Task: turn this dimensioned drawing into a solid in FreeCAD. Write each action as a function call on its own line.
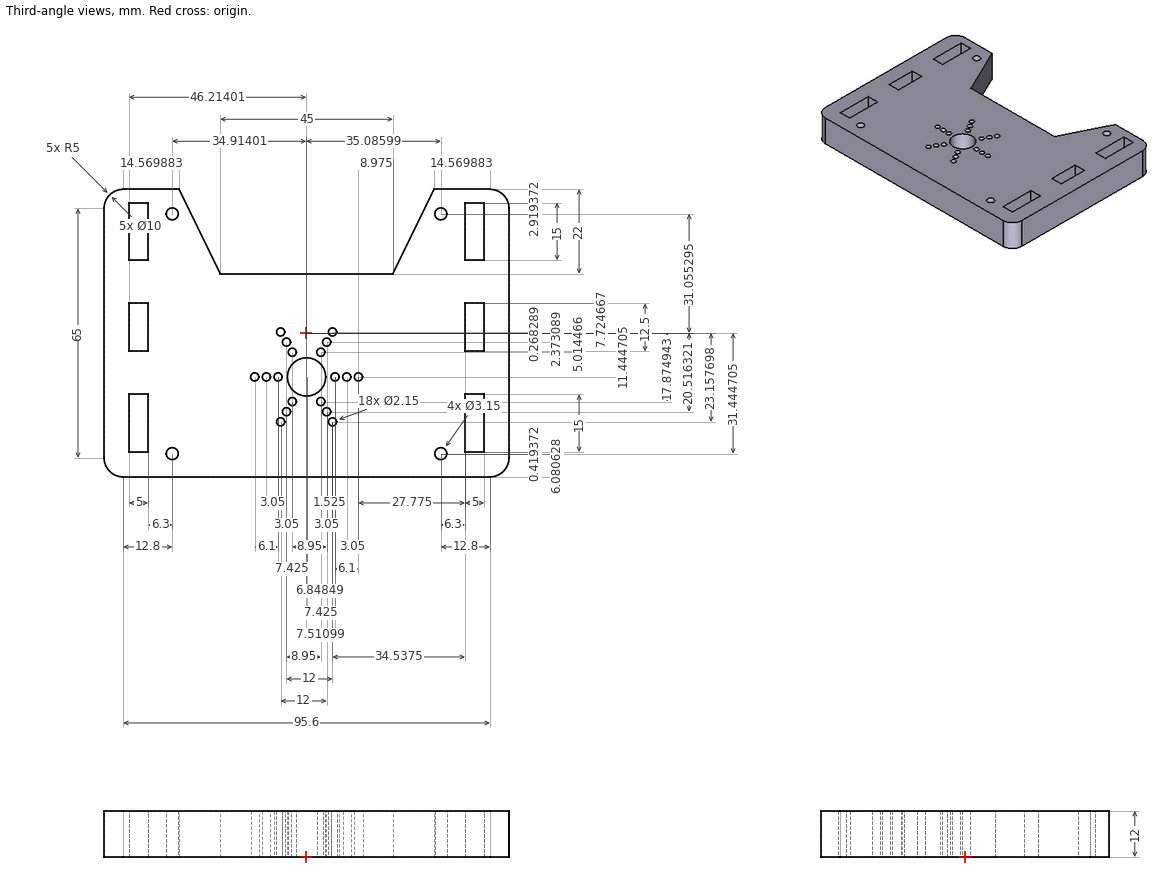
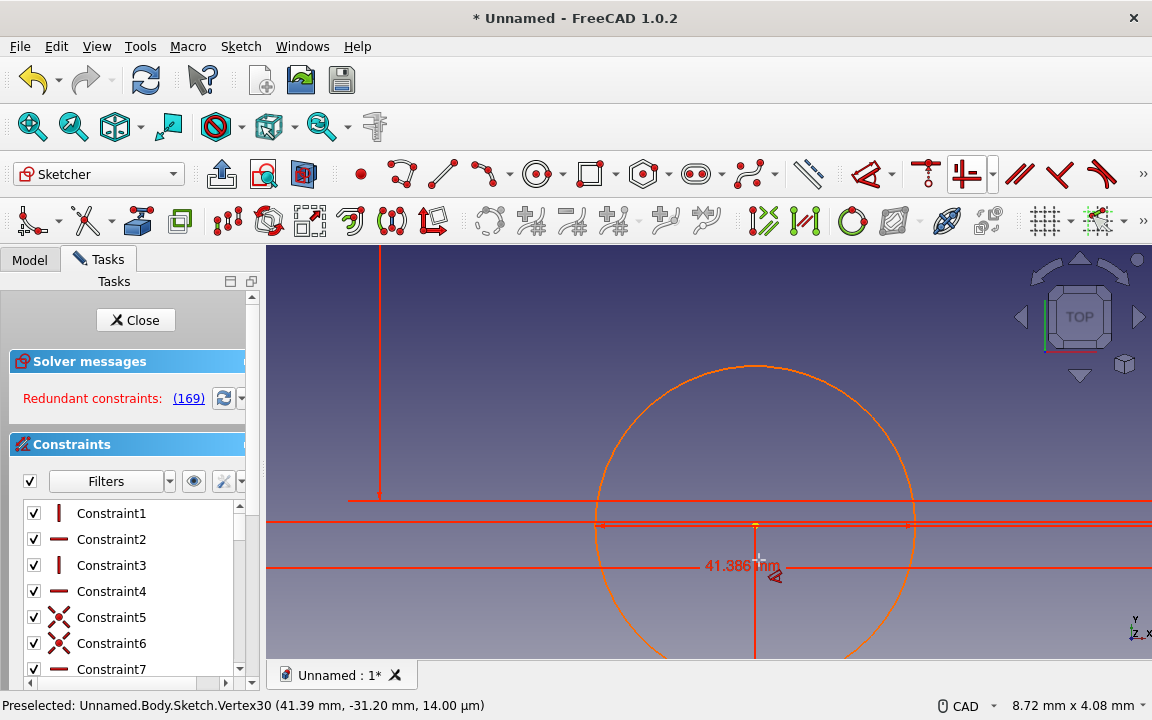
click(755, 526)
click(721, 514)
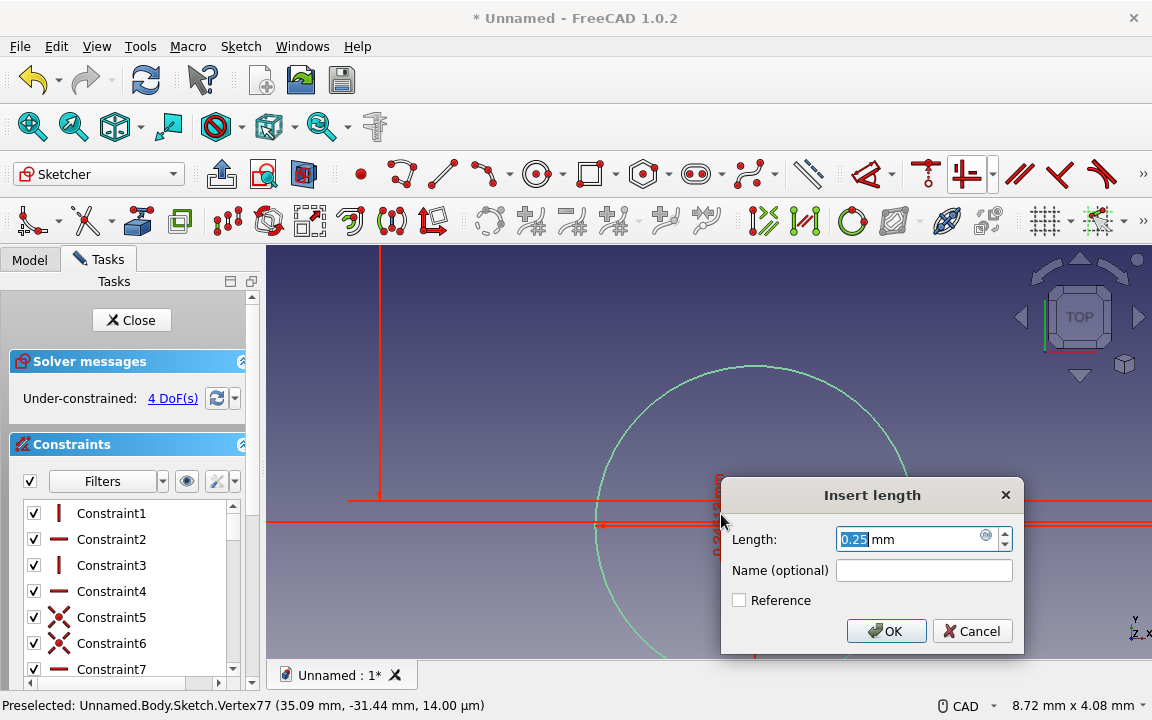
text(0.419372)
key(Return)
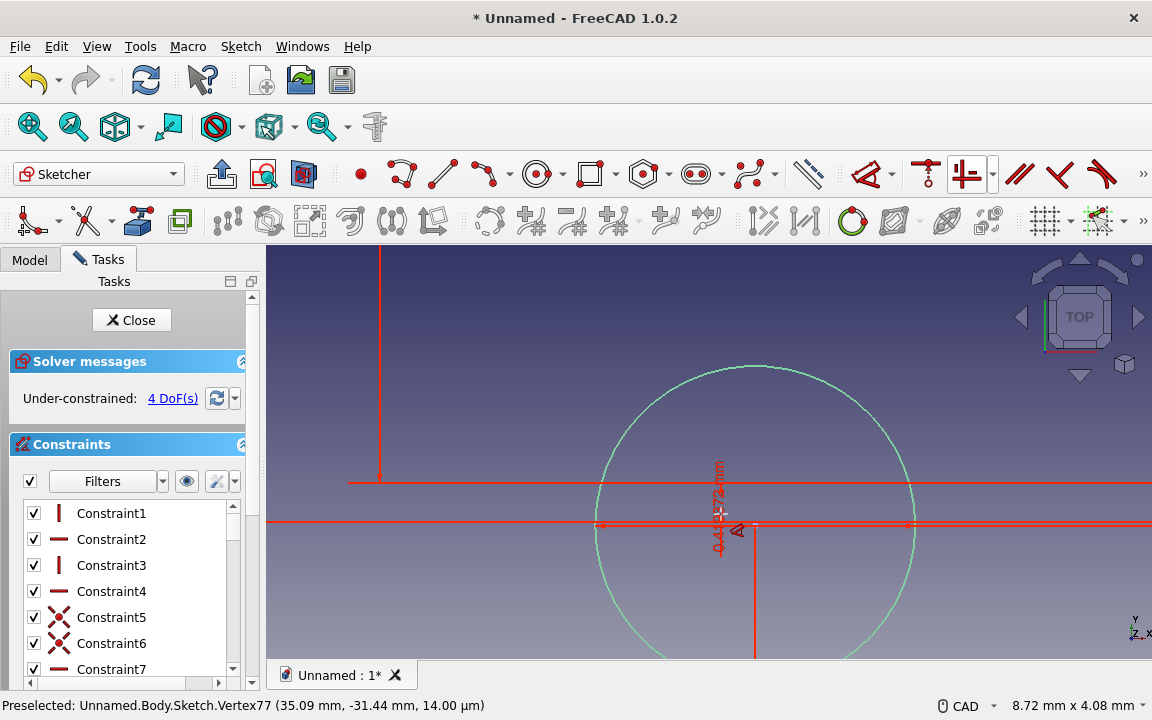
scroll(759, 560, down, 17)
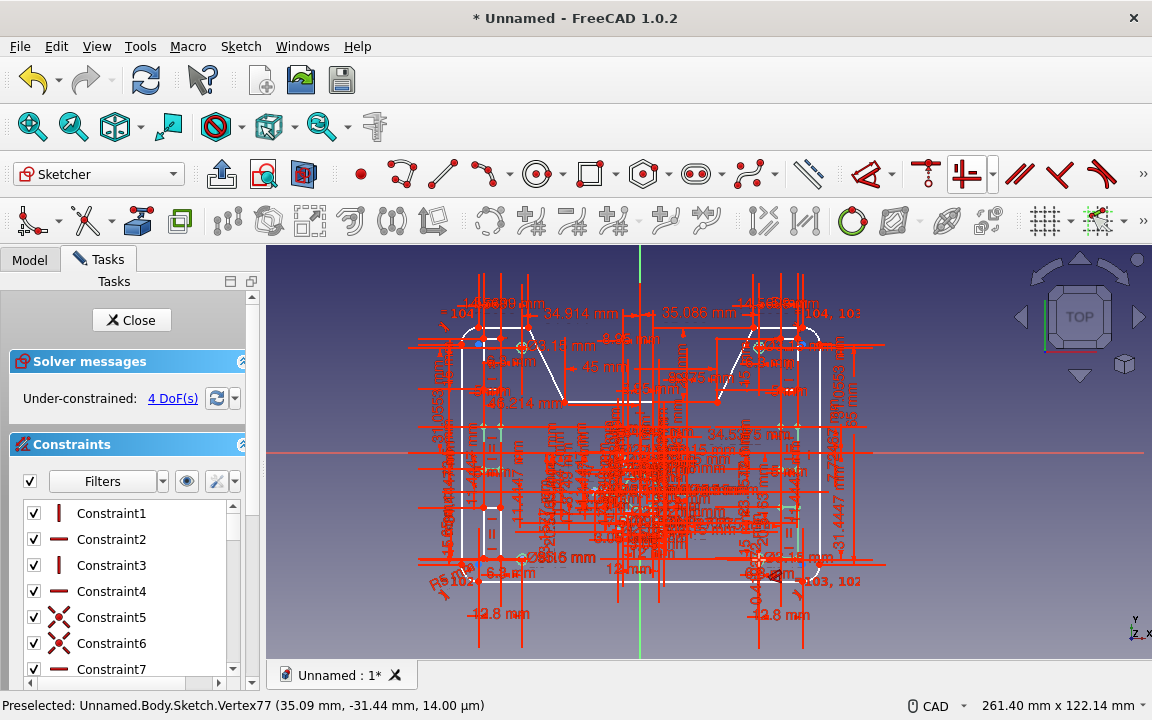
scroll(803, 582, up, 4)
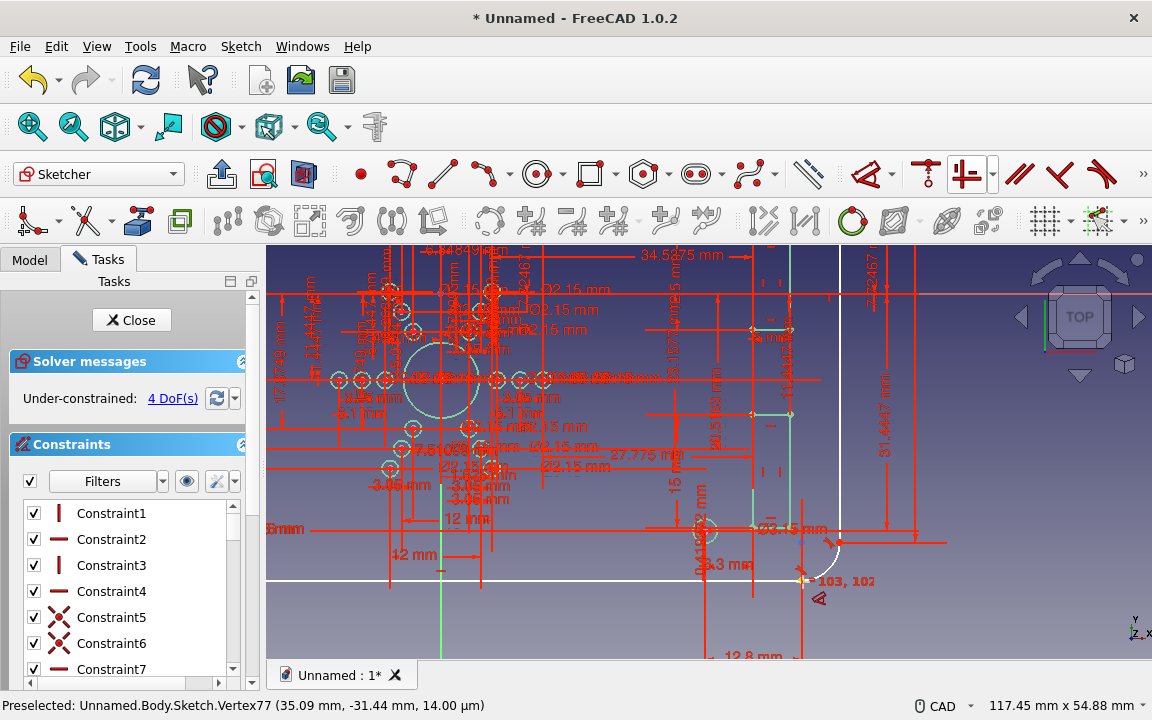
click(802, 581)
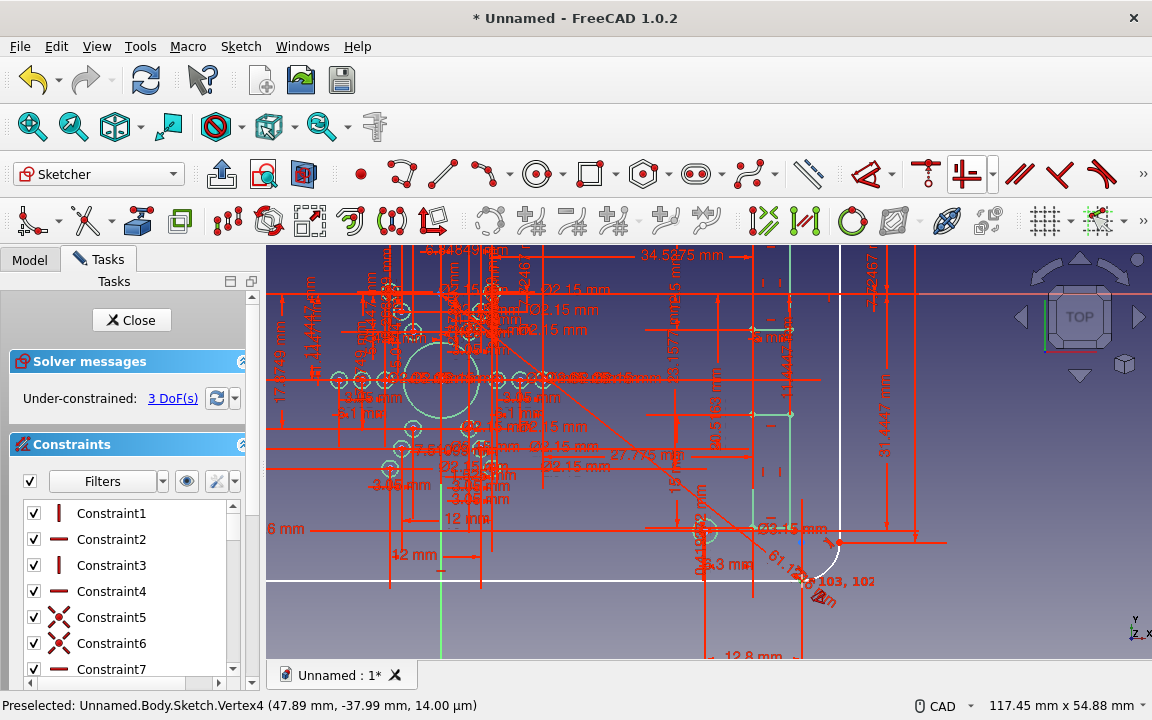
click(705, 531)
click(860, 556)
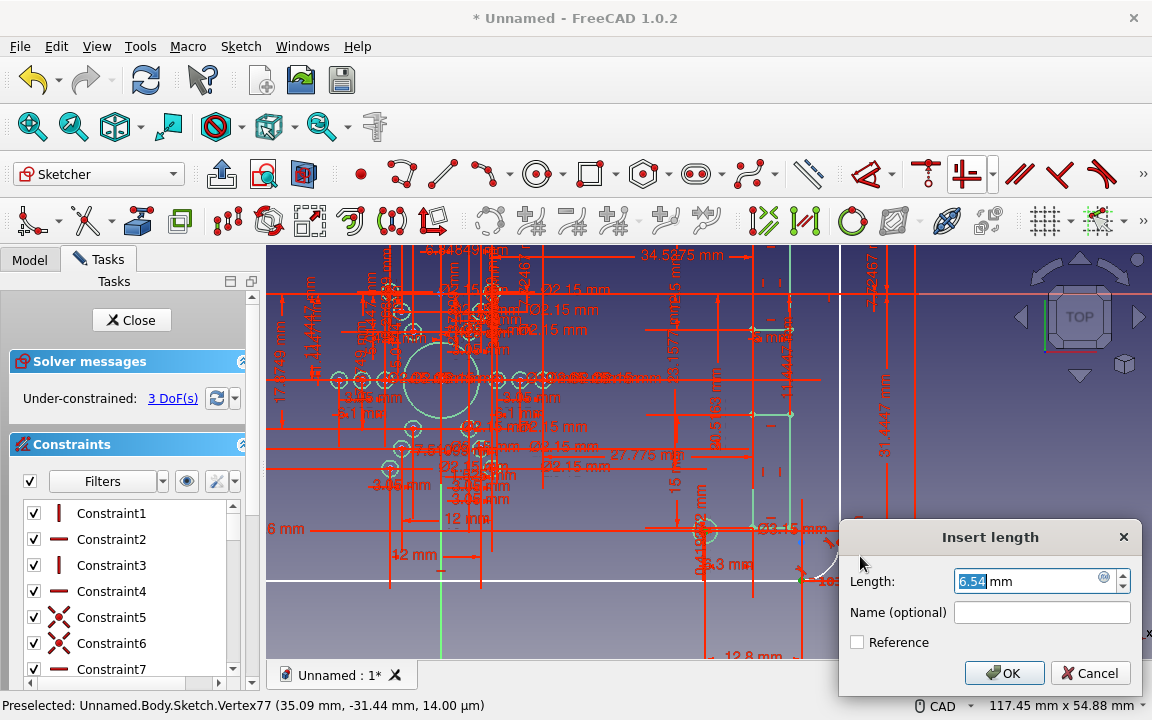
text(6.080628)
key(Return)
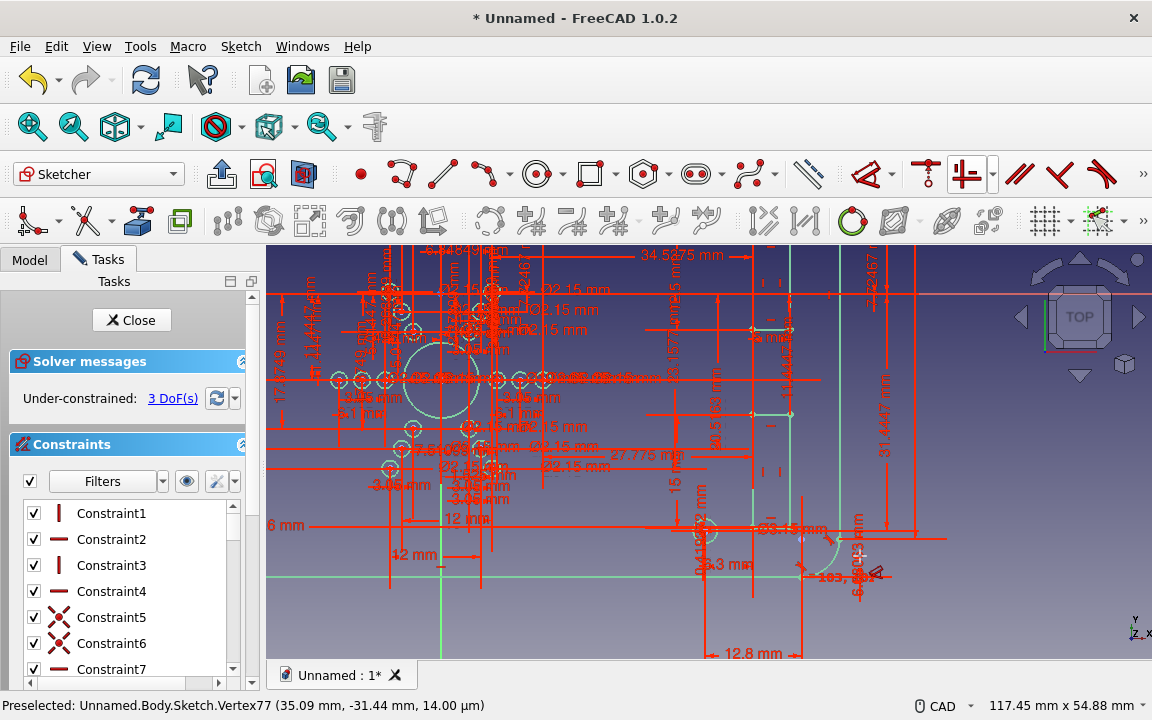
scroll(803, 581, down, 4)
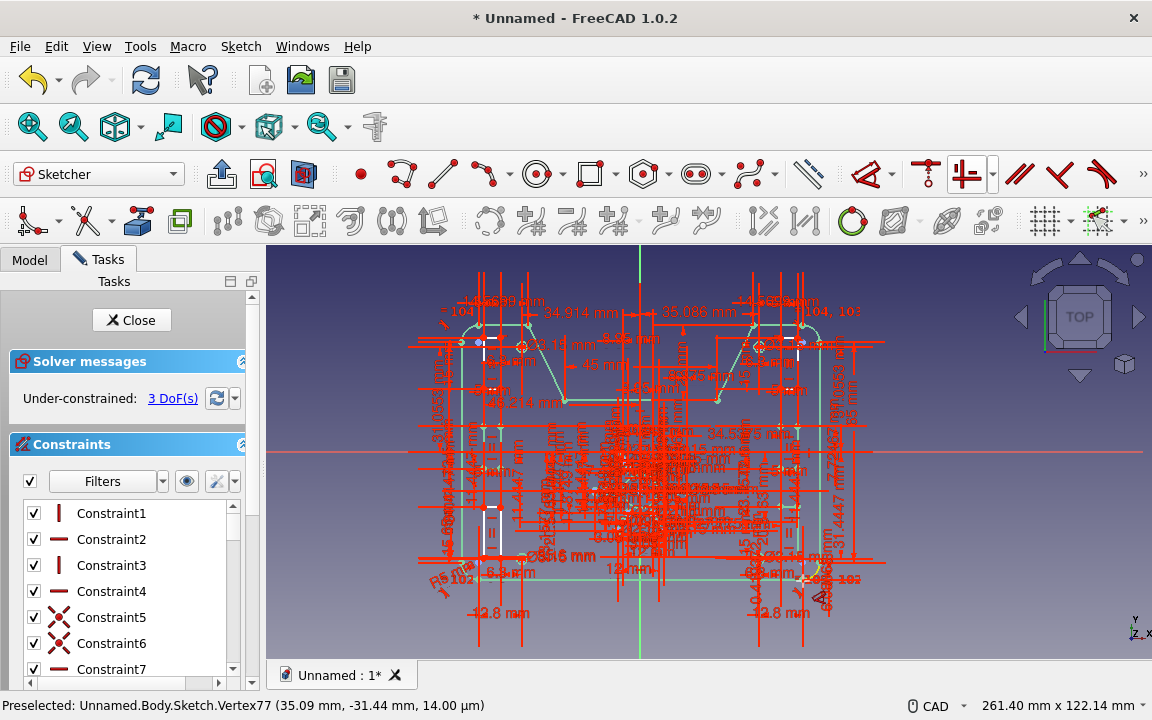
scroll(501, 558, up, 17)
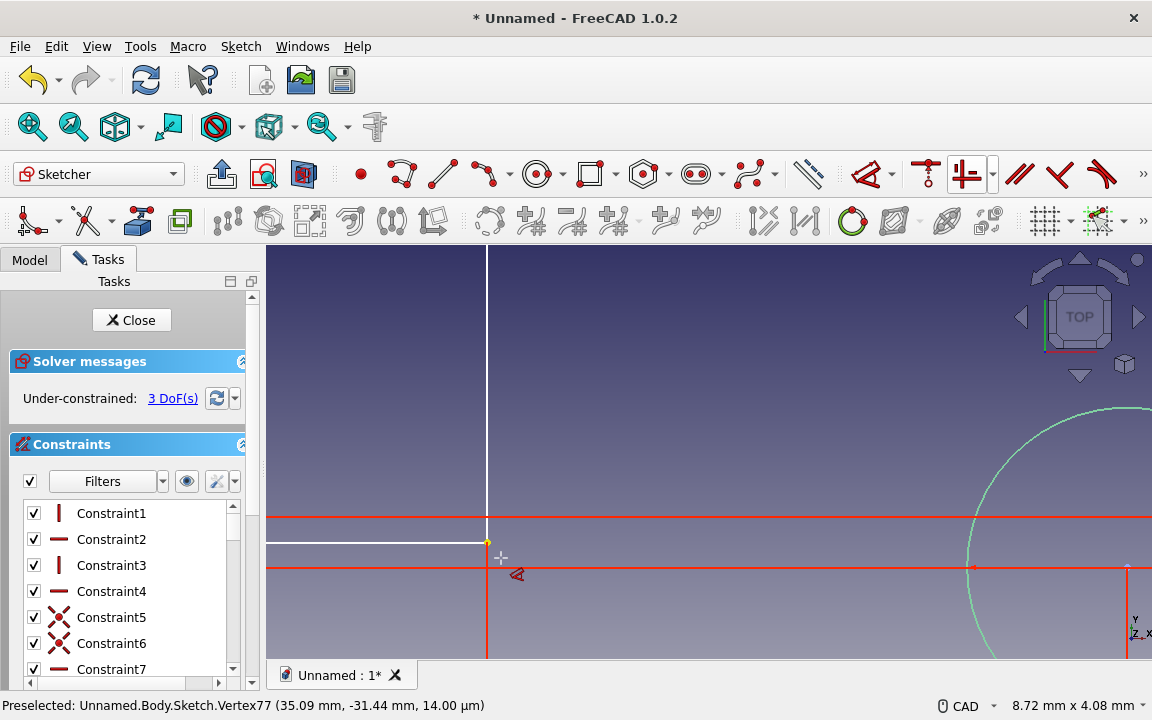
click(487, 543)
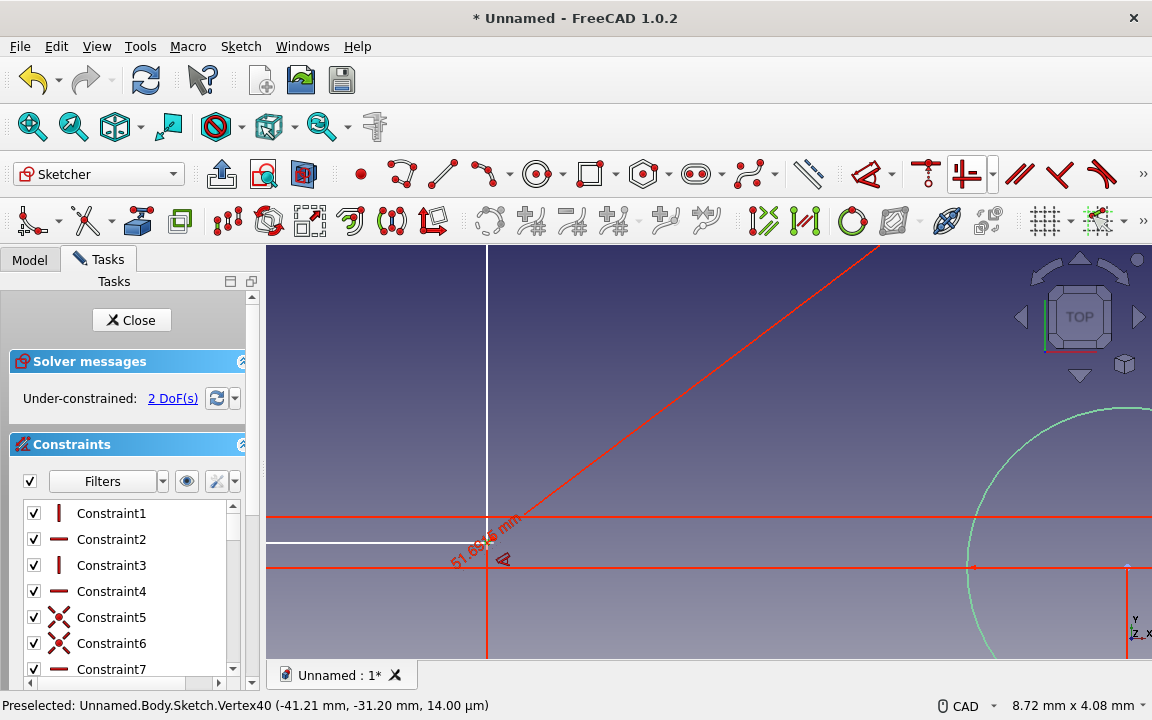
scroll(501, 558, down, 17)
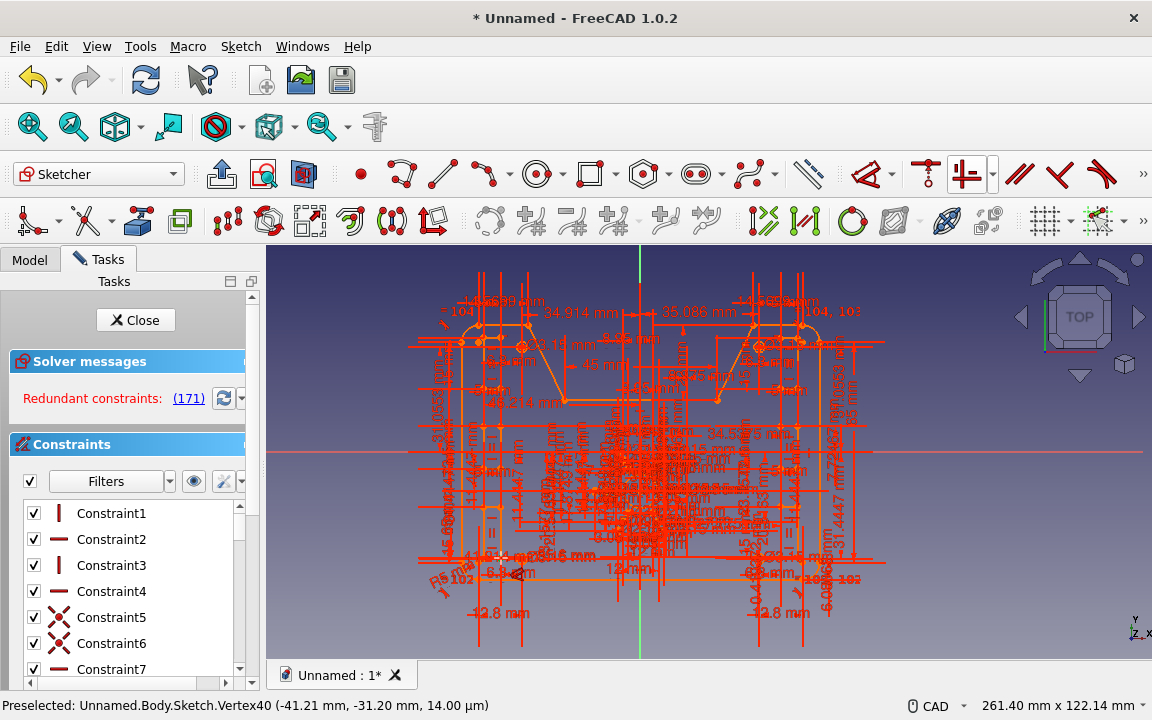
scroll(522, 559, up, 17)